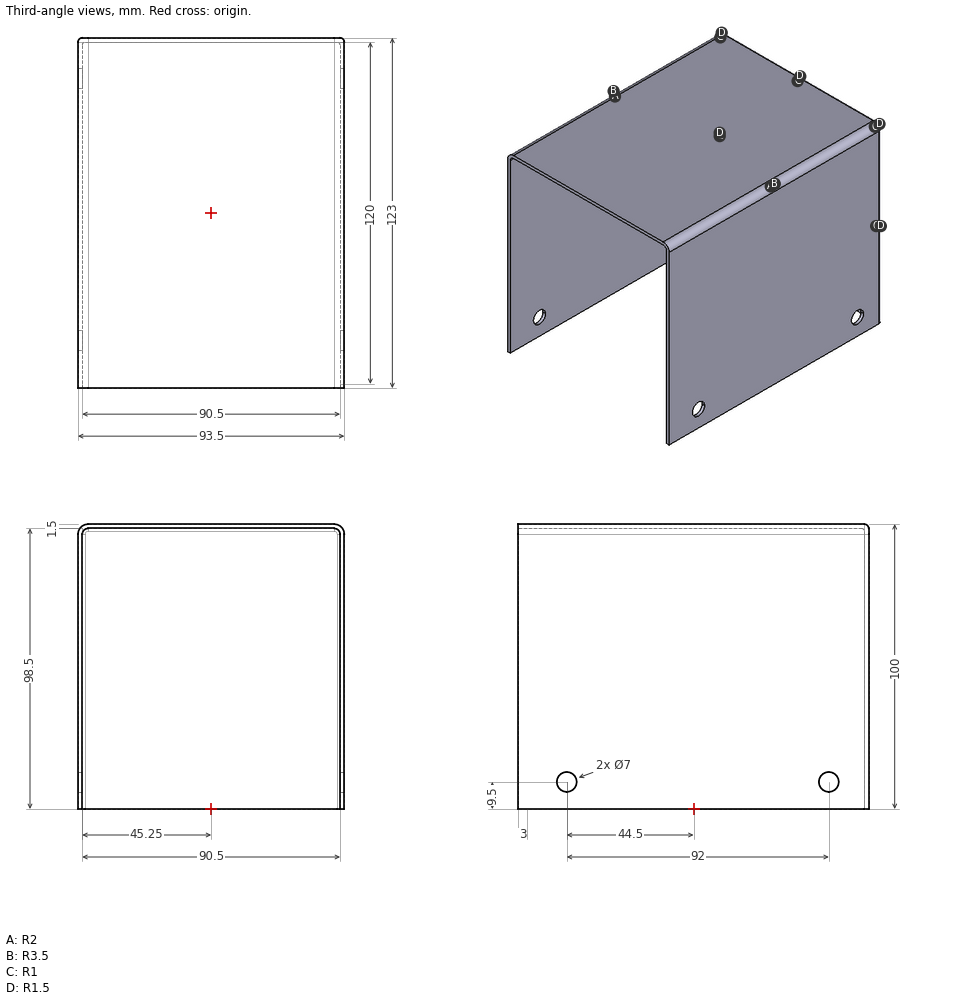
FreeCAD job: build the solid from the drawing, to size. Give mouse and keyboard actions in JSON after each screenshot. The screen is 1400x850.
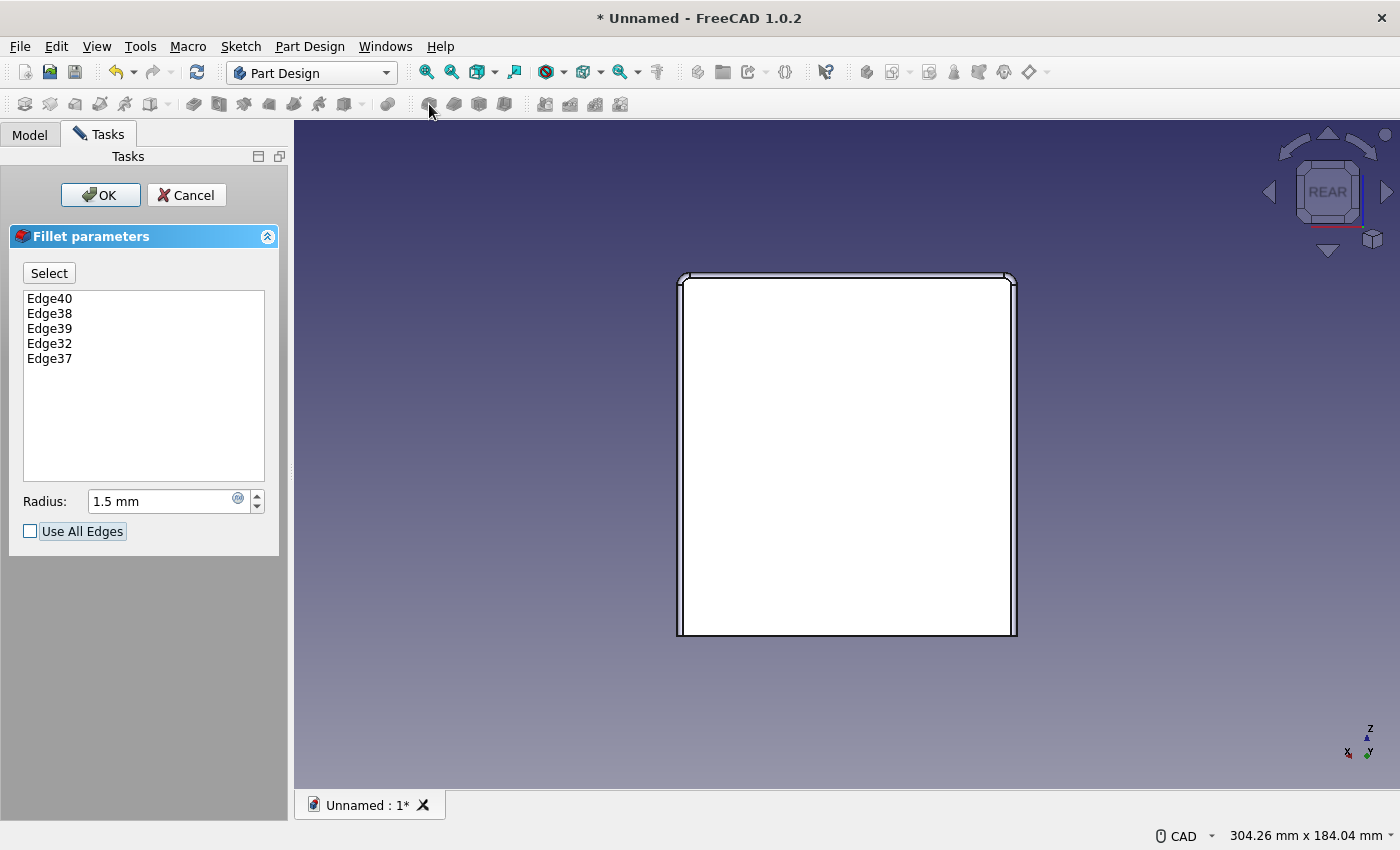
{"action": "left_click", "coordinate": [101, 195]}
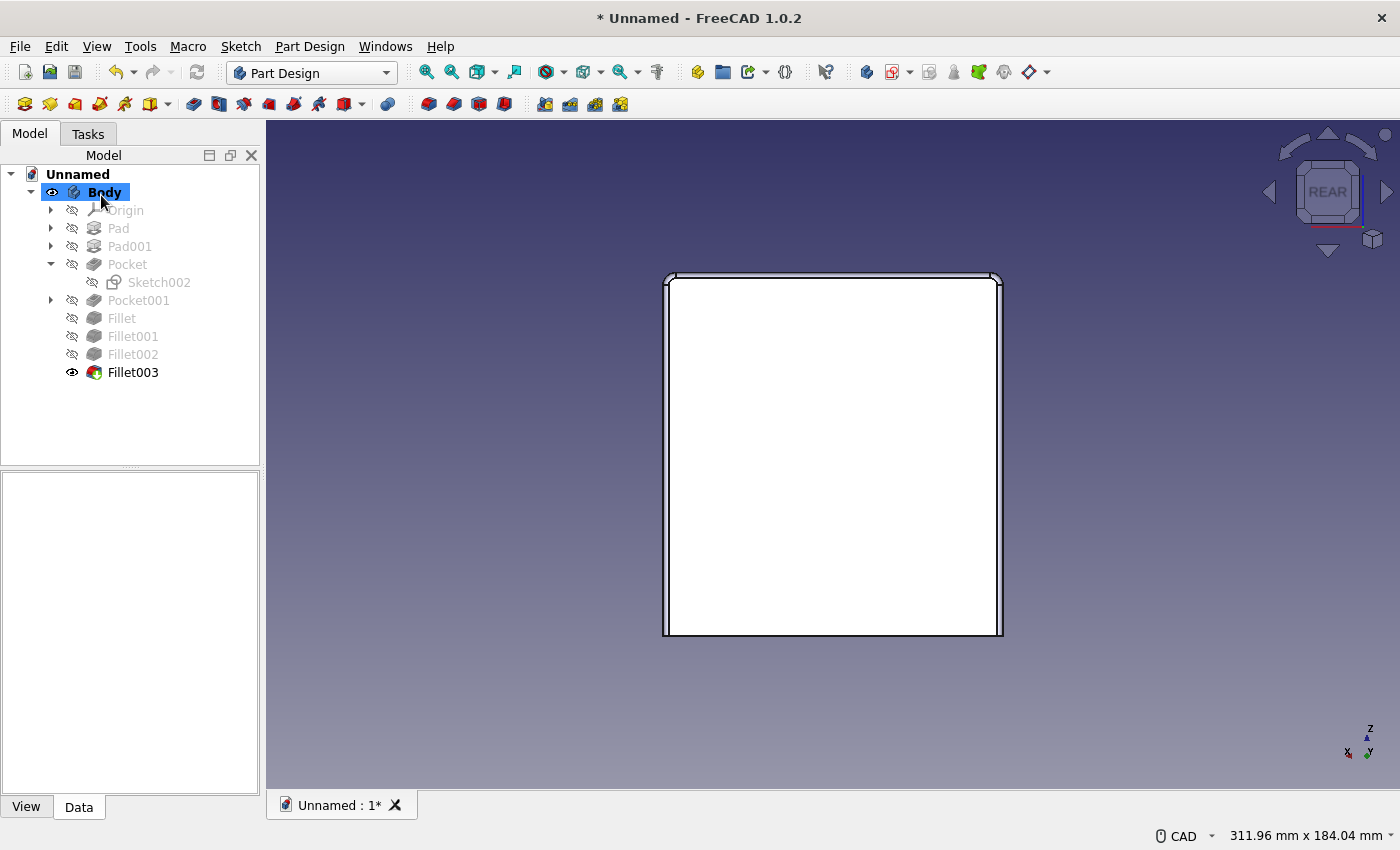
{"action": "key", "text": "0"}